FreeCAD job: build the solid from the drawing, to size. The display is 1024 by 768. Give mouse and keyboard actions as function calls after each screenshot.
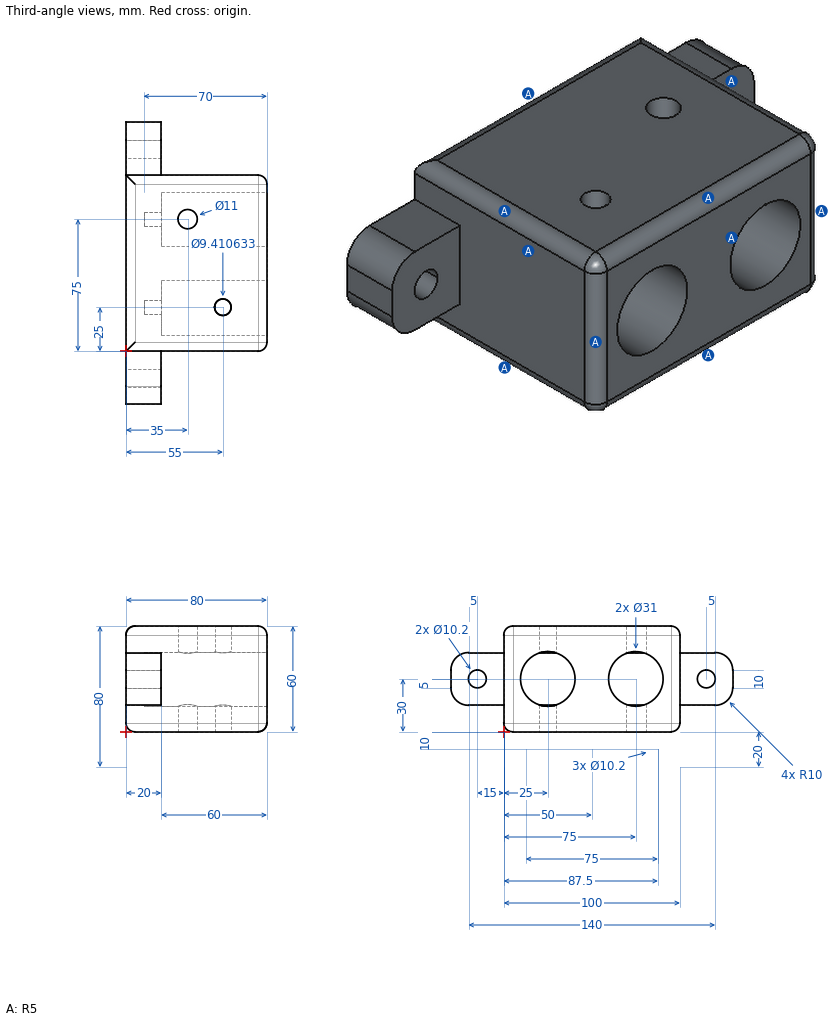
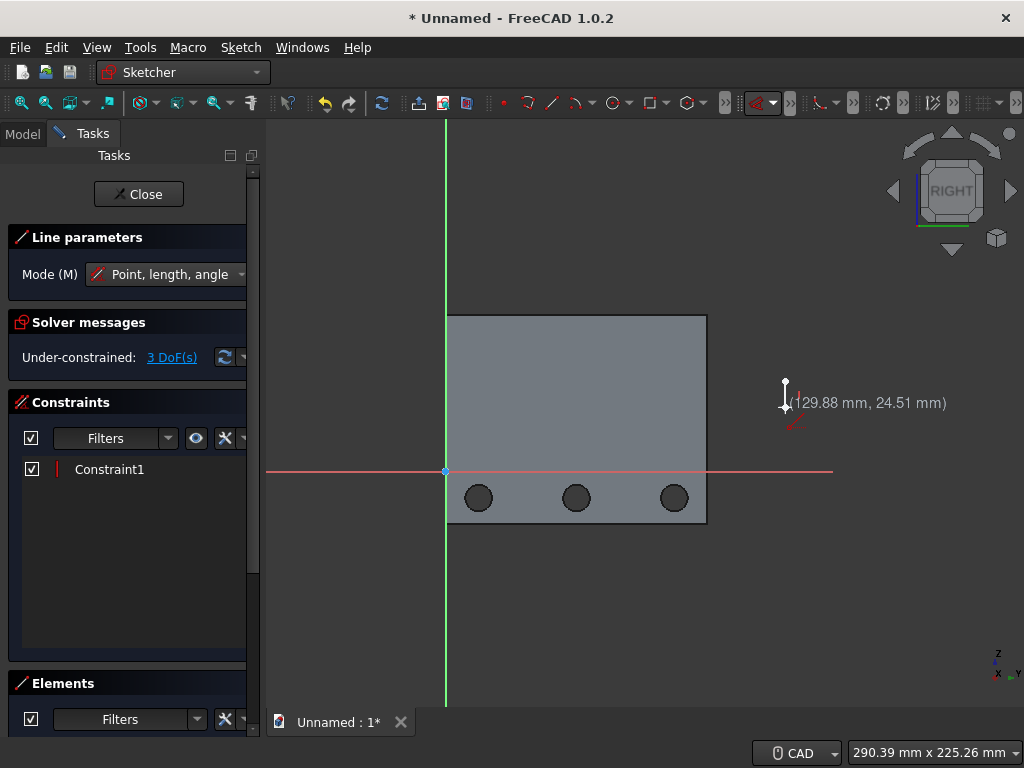
click(759, 433)
click(394, 433)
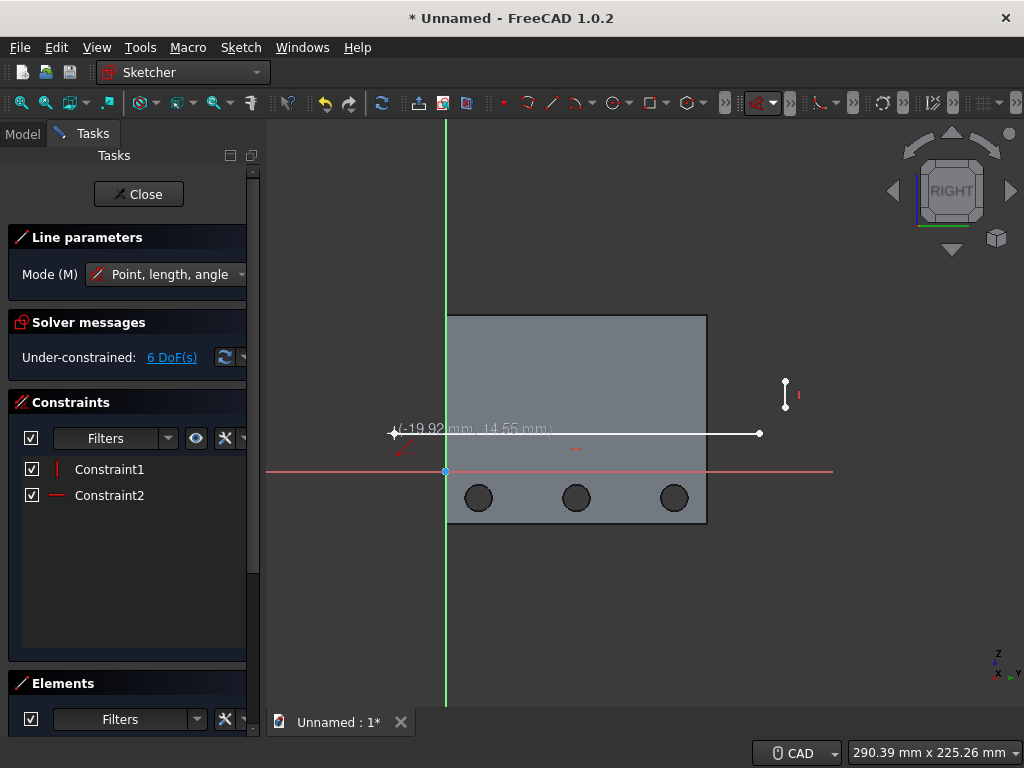
click(368, 407)
click(368, 381)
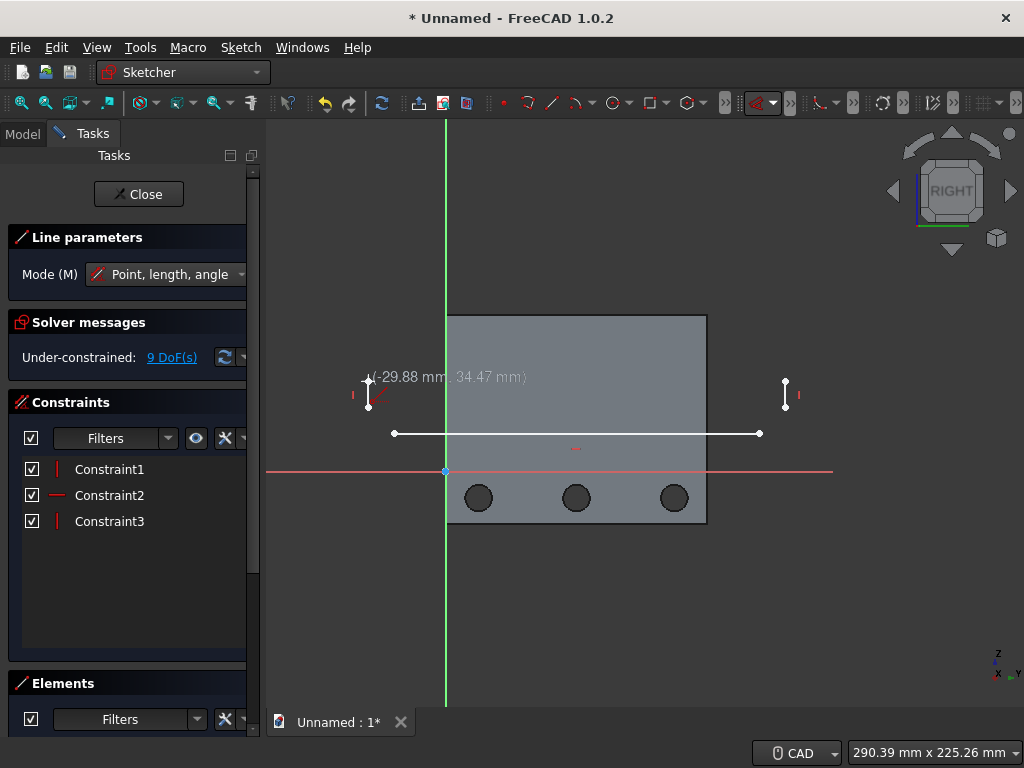
click(394, 355)
click(759, 355)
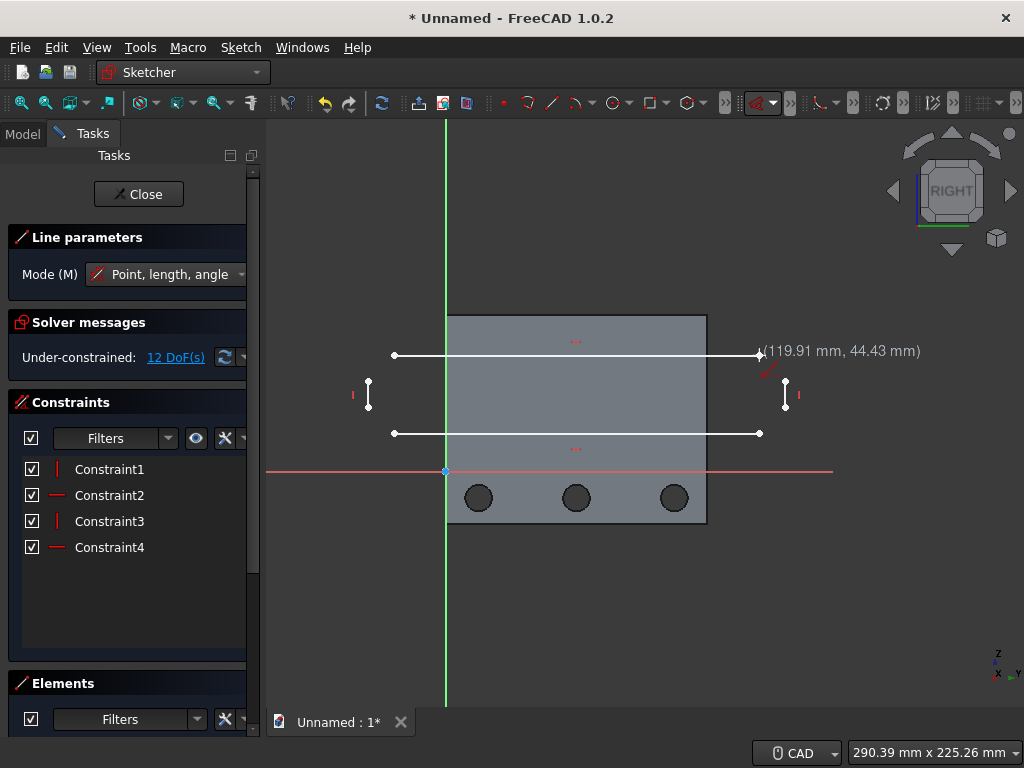
key(g)
key(3)
key(a)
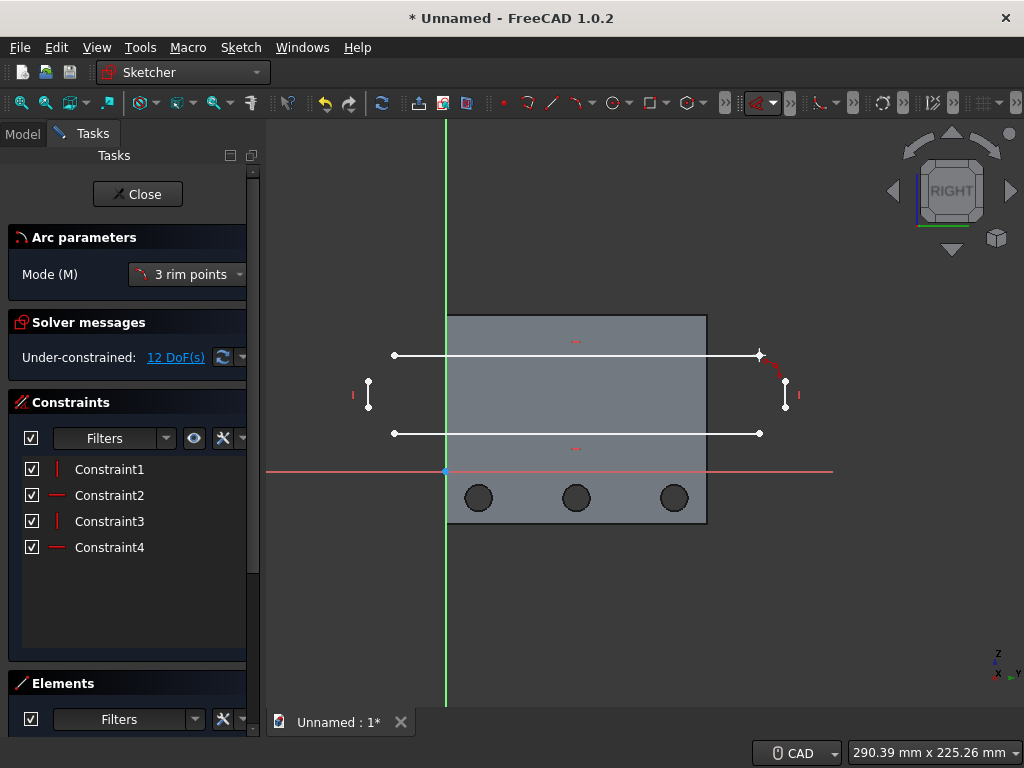
click(785, 408)
click(759, 434)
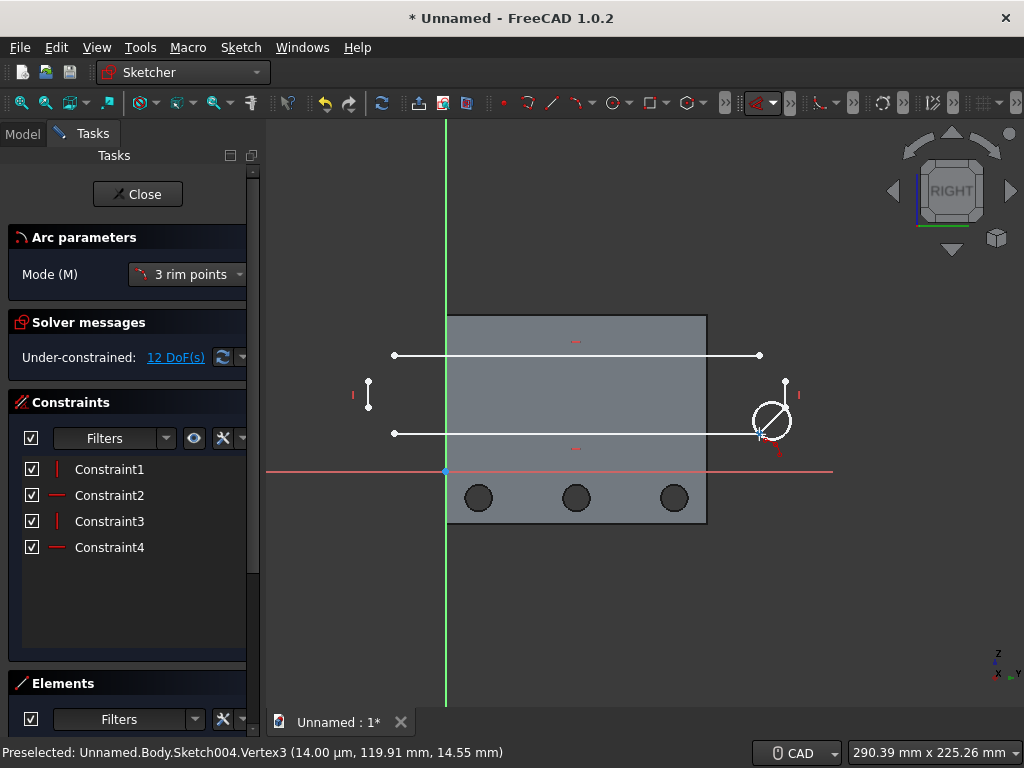
scroll(778, 425, up, 4)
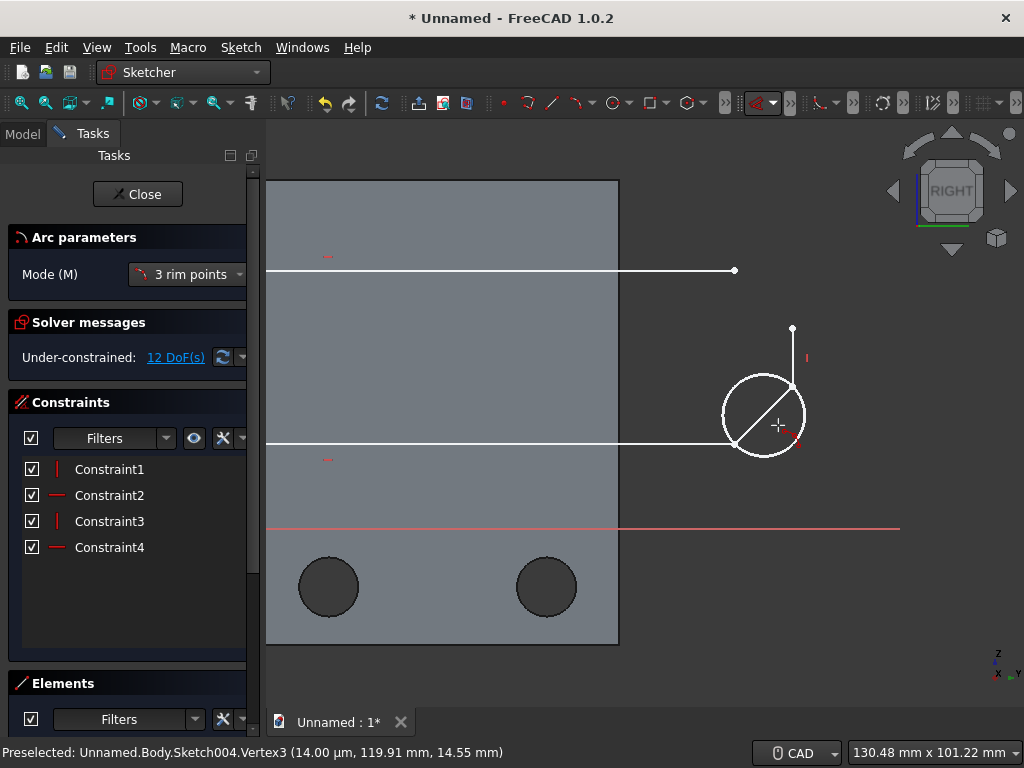
click(776, 425)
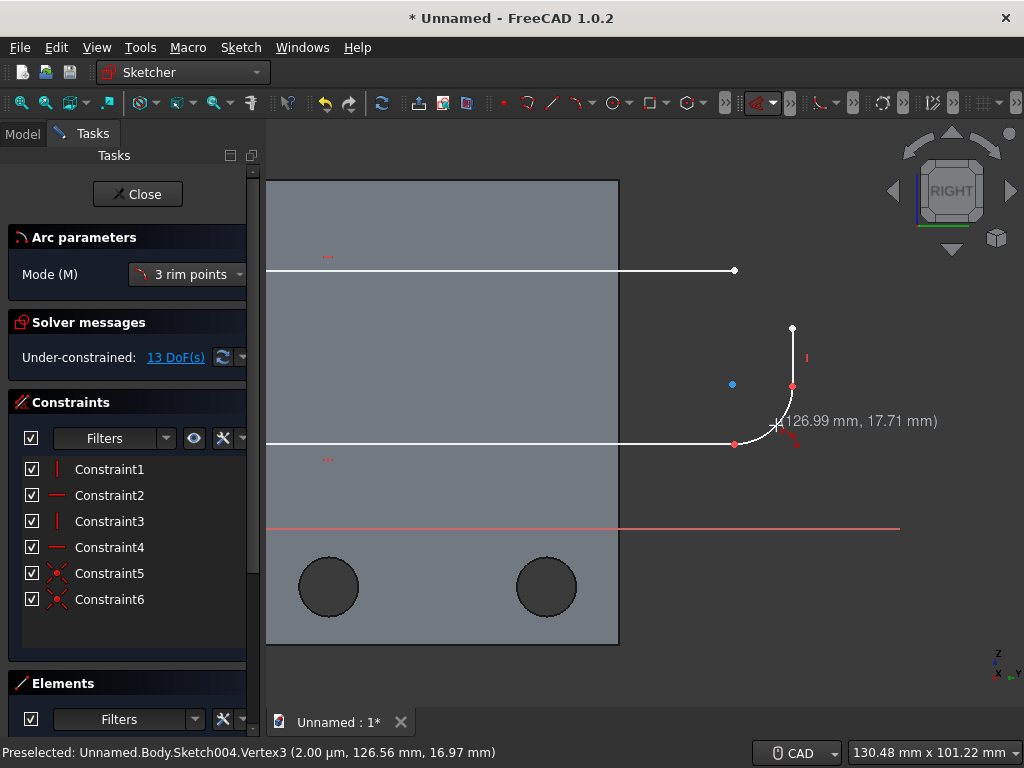
scroll(779, 425, down, 4)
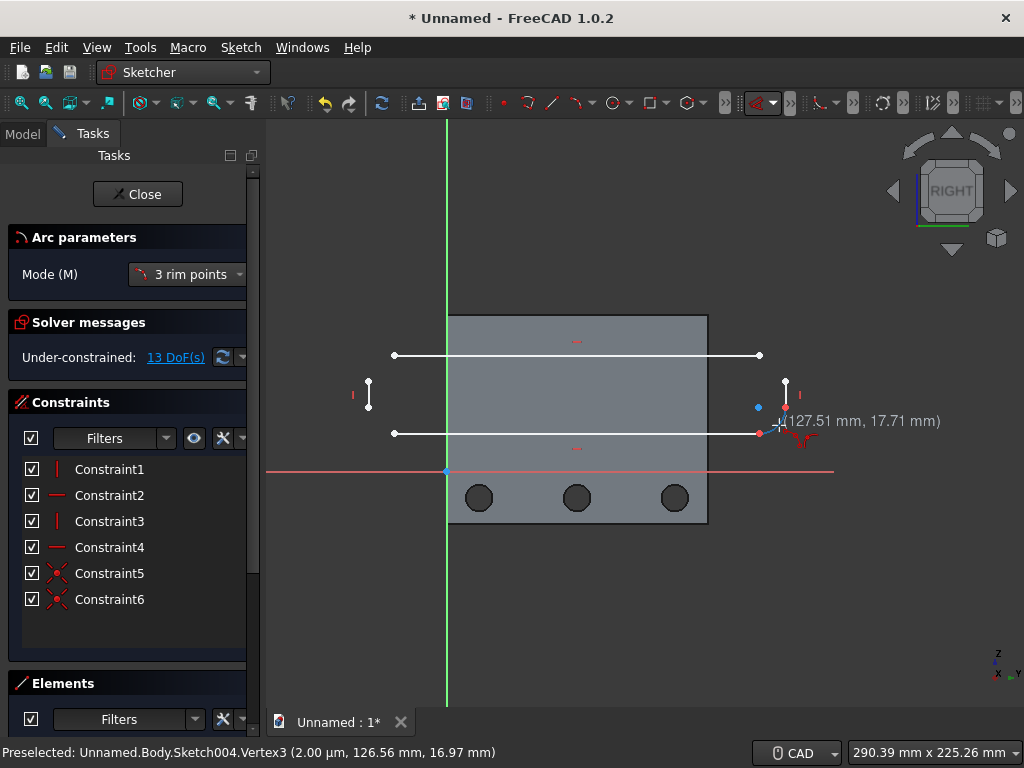
click(395, 434)
click(369, 408)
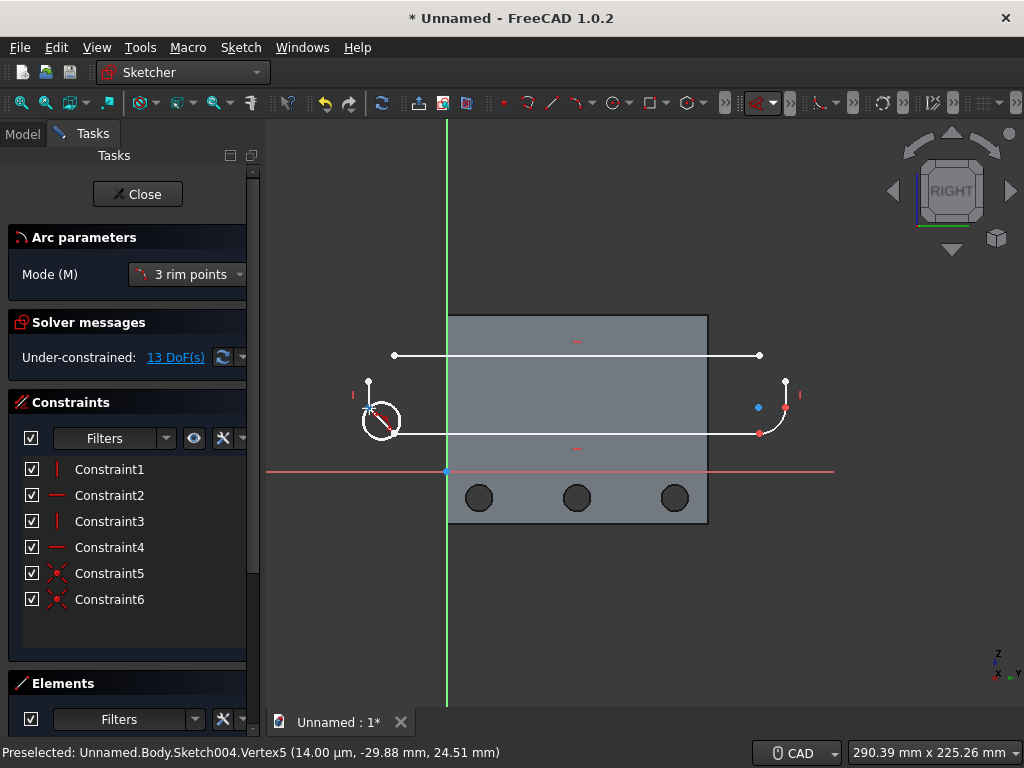
scroll(376, 425, up, 4)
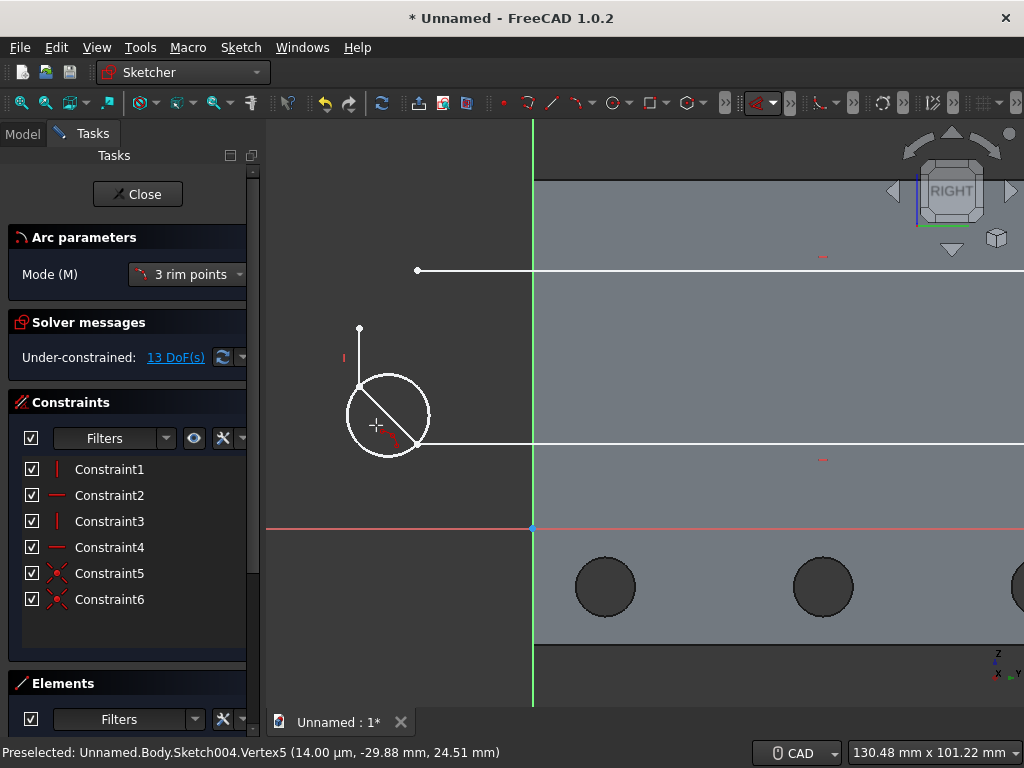
click(376, 425)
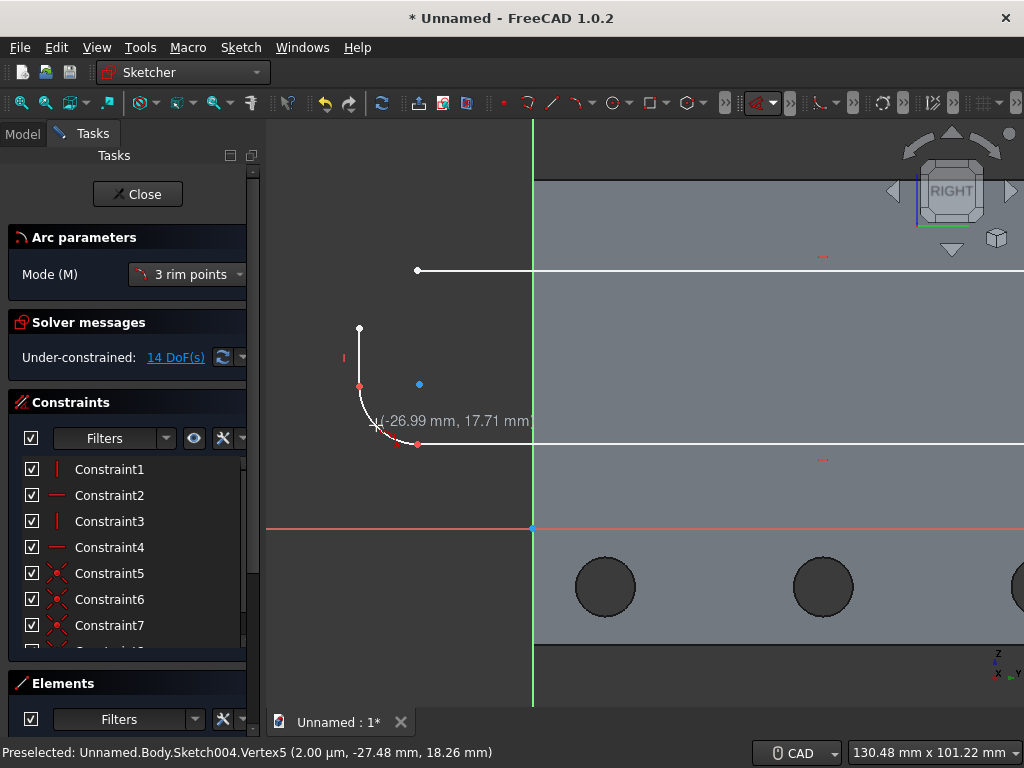
click(359, 329)
click(417, 271)
click(376, 285)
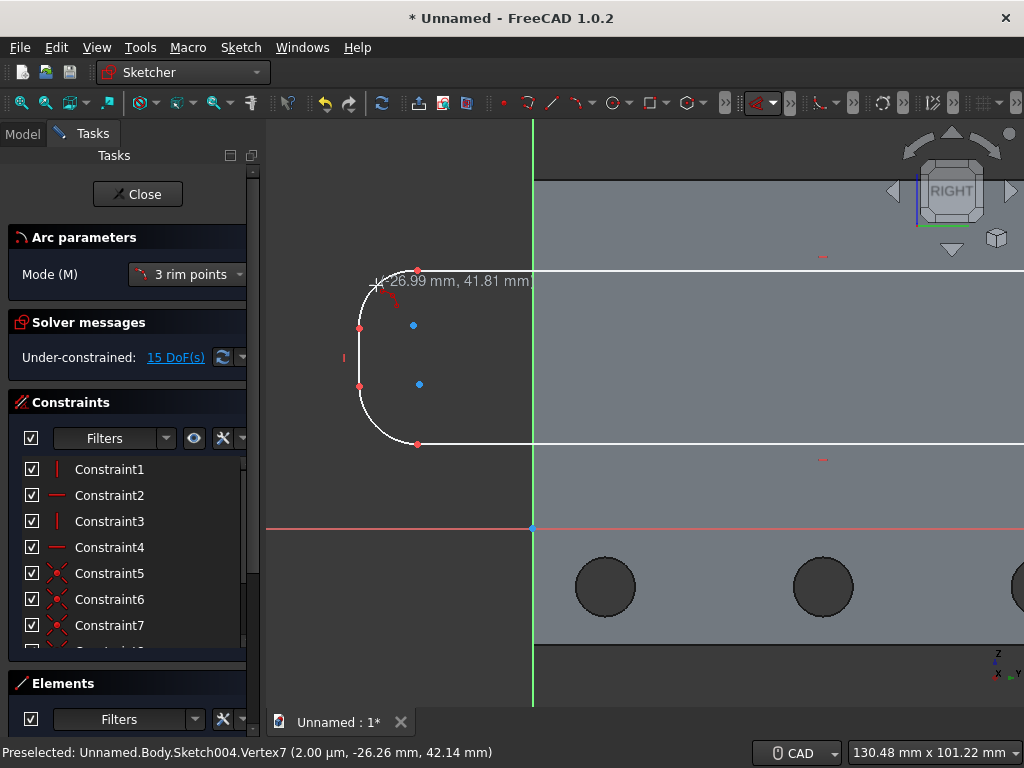
scroll(375, 425, down, 4)